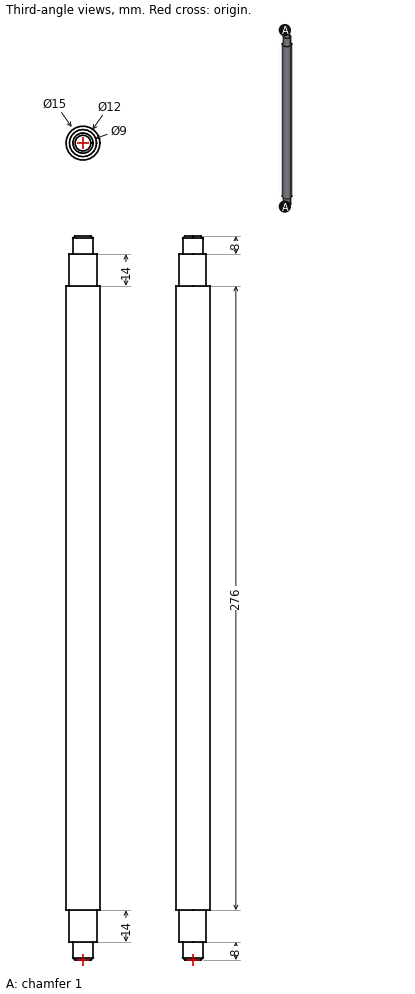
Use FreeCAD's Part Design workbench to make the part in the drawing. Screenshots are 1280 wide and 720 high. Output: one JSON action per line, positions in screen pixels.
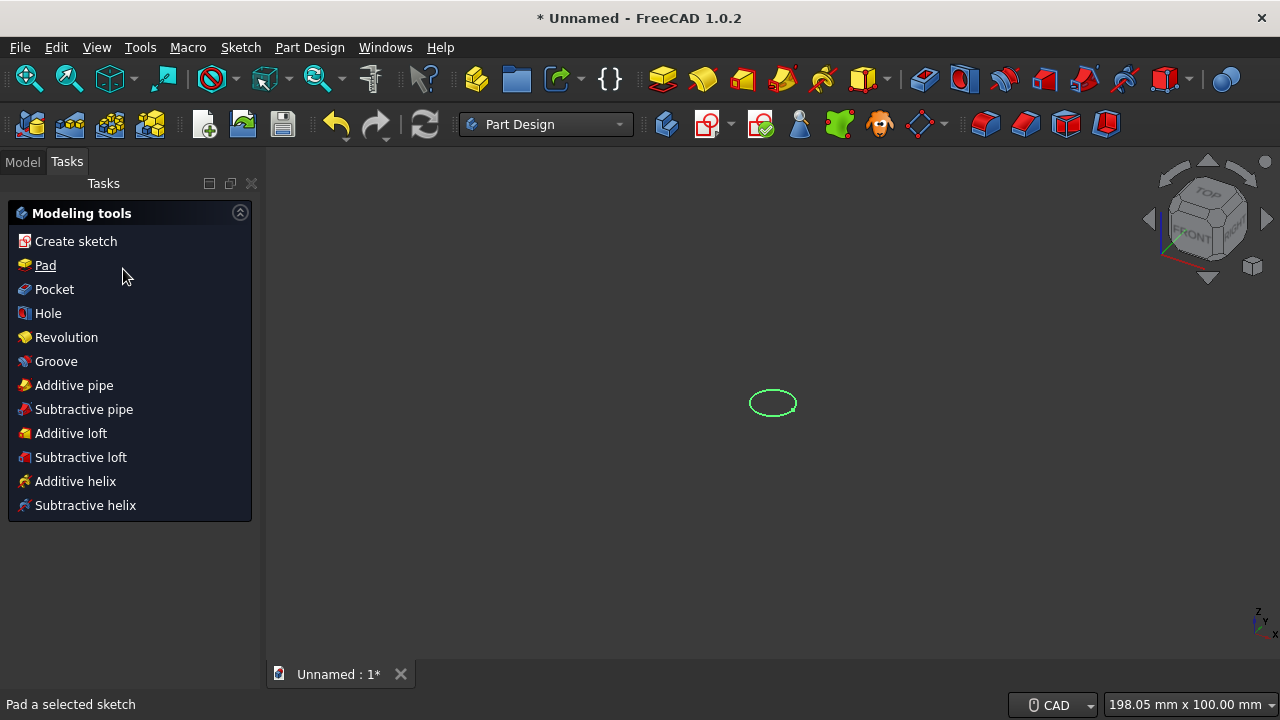
{"action": "left_click", "coordinate": [664, 80]}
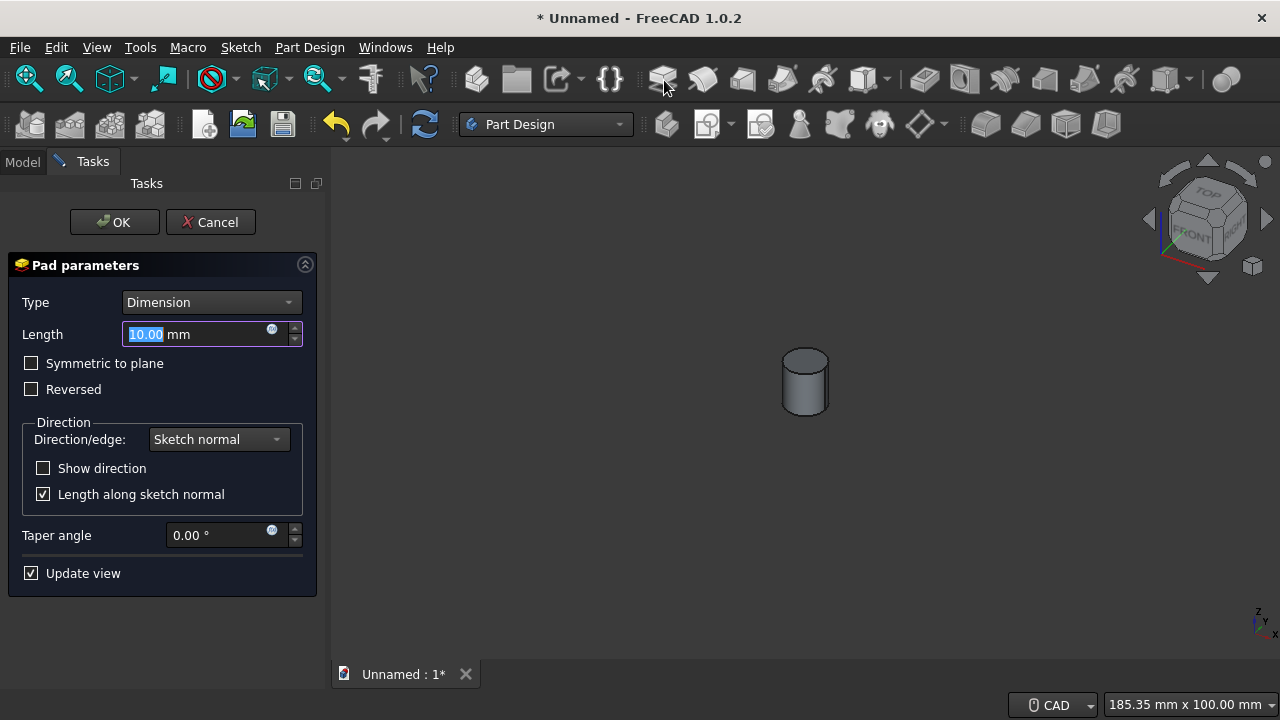
{"action": "type", "text": "8"}
{"action": "key", "text": "Tab"}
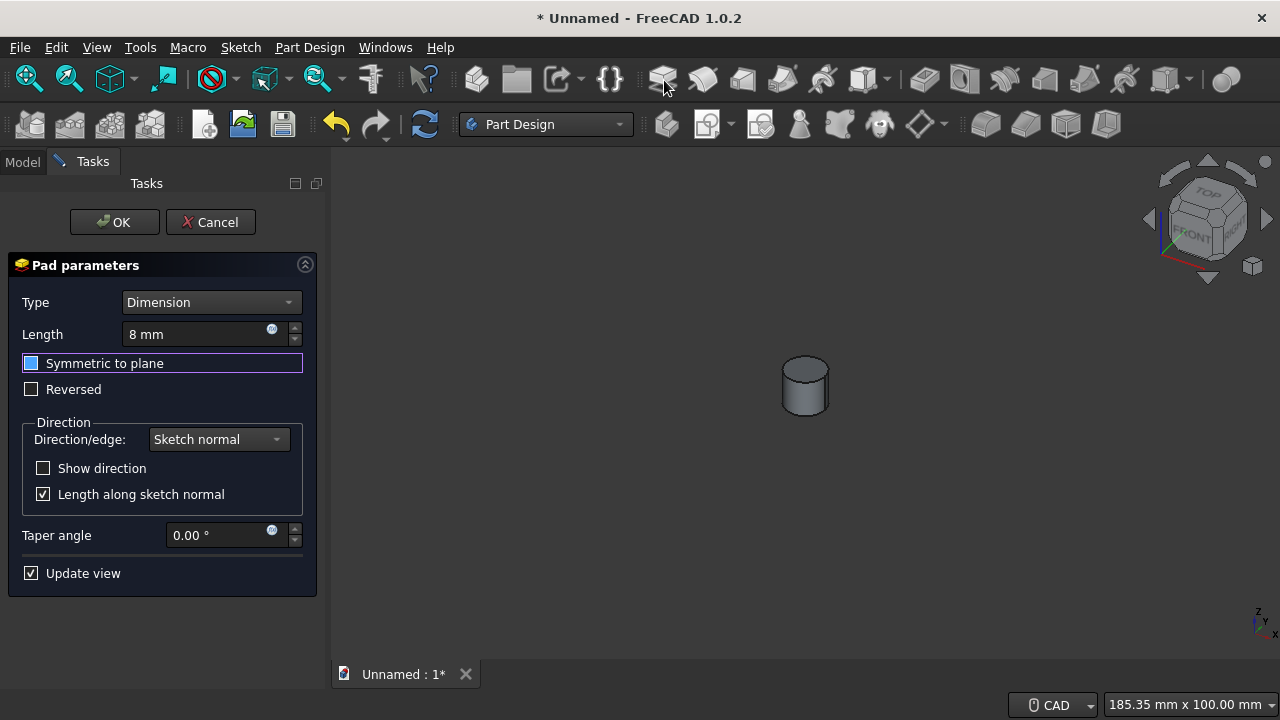
{"action": "left_click", "coordinate": [115, 222]}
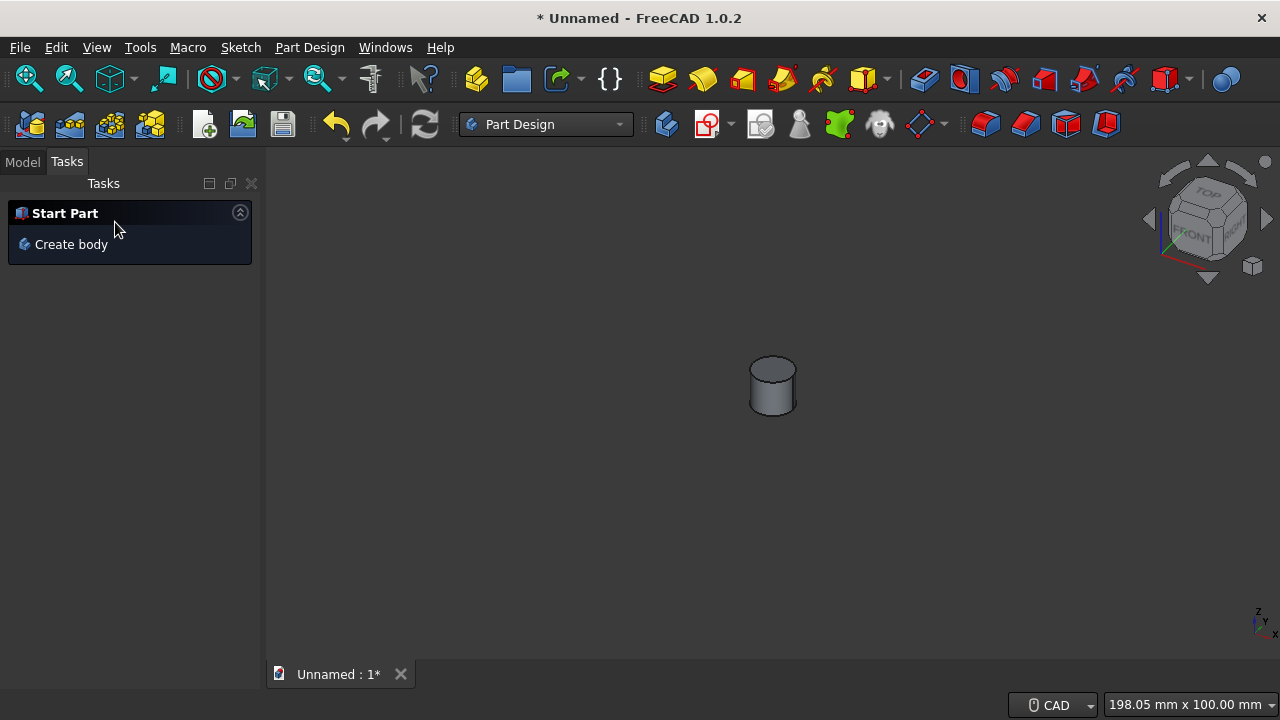
{"action": "key", "text": "v f"}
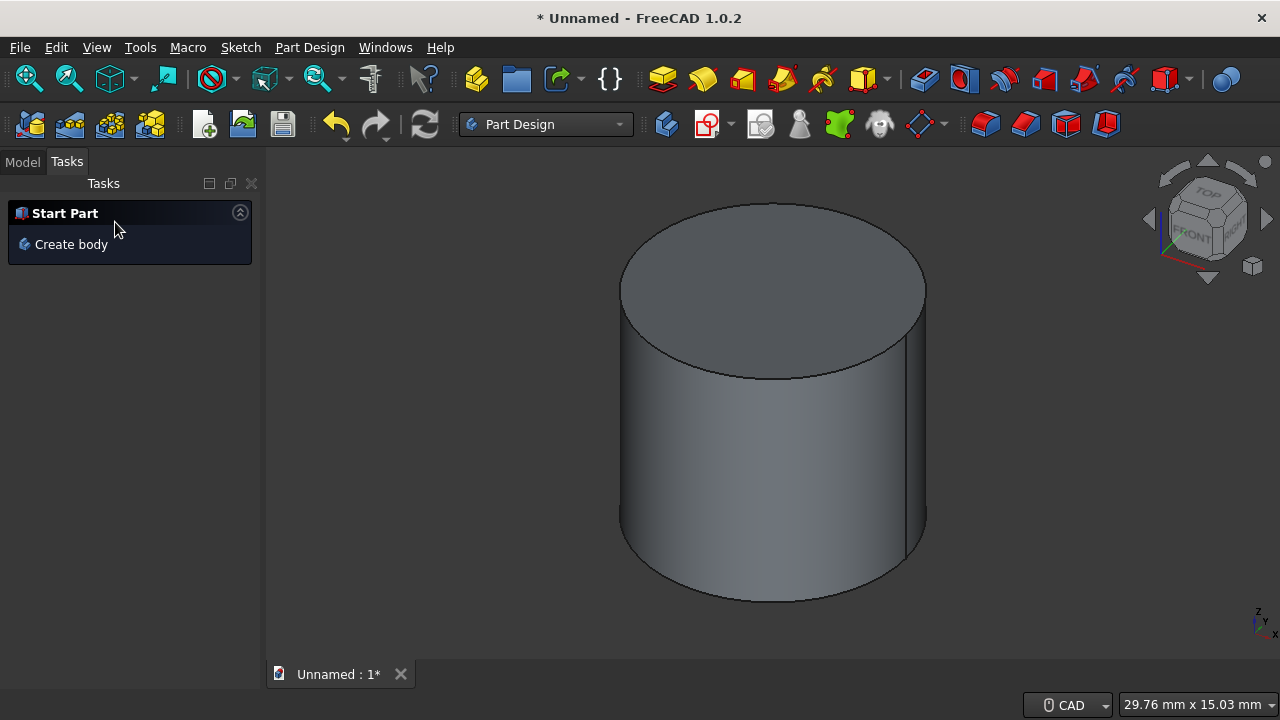
{"action": "left_click", "coordinate": [773, 290]}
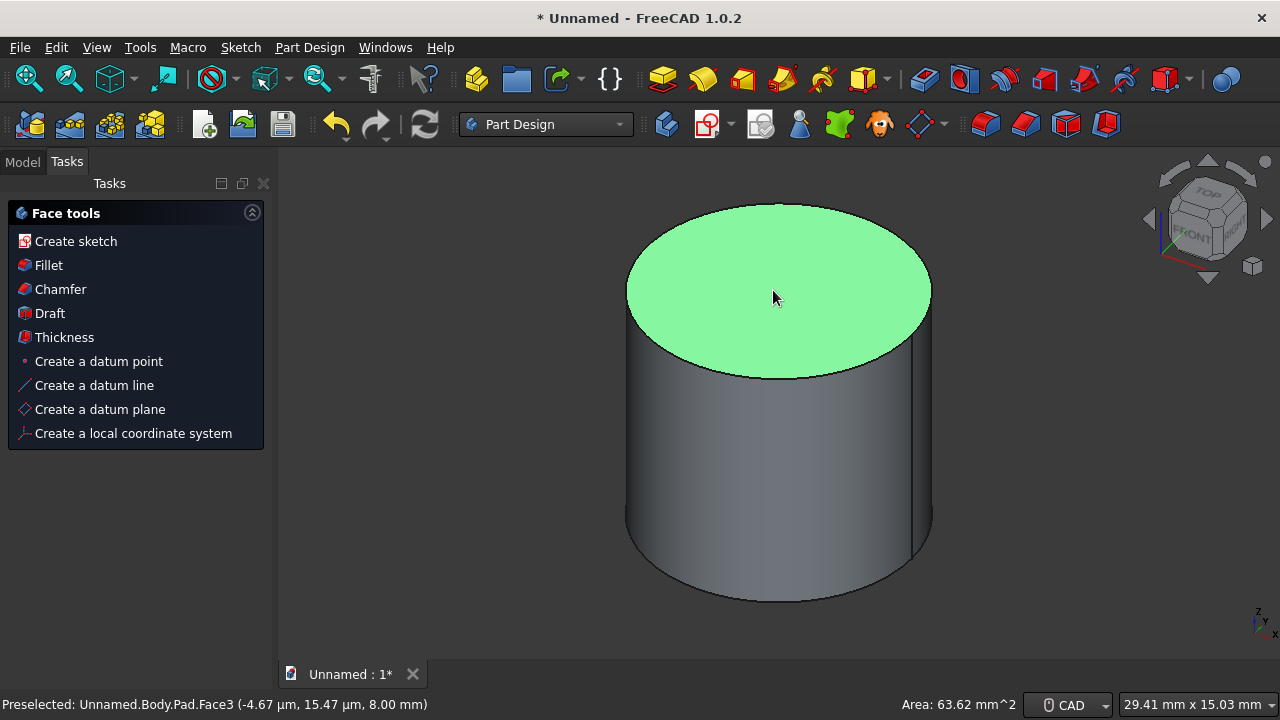
{"action": "left_click", "coordinate": [708, 124]}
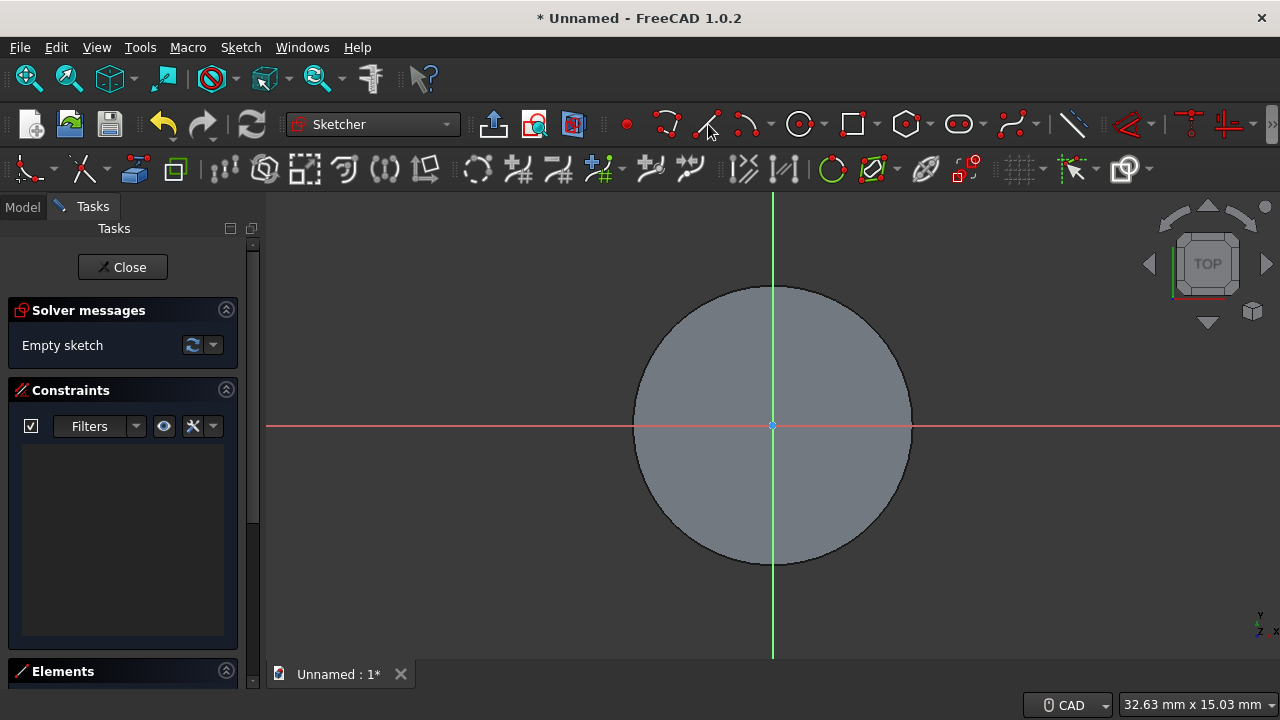
{"action": "scroll", "coordinate": [396, 425], "scroll_direction": "down", "scroll_amount": 1}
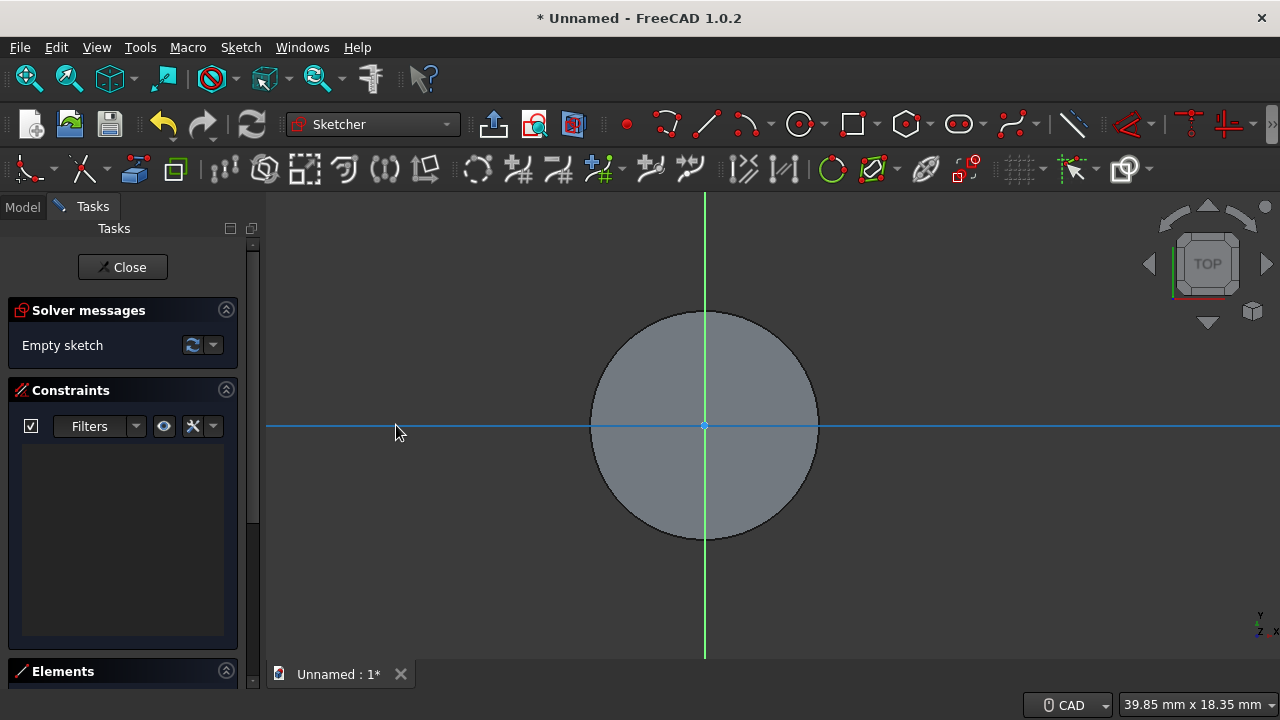
{"action": "key", "text": "g c"}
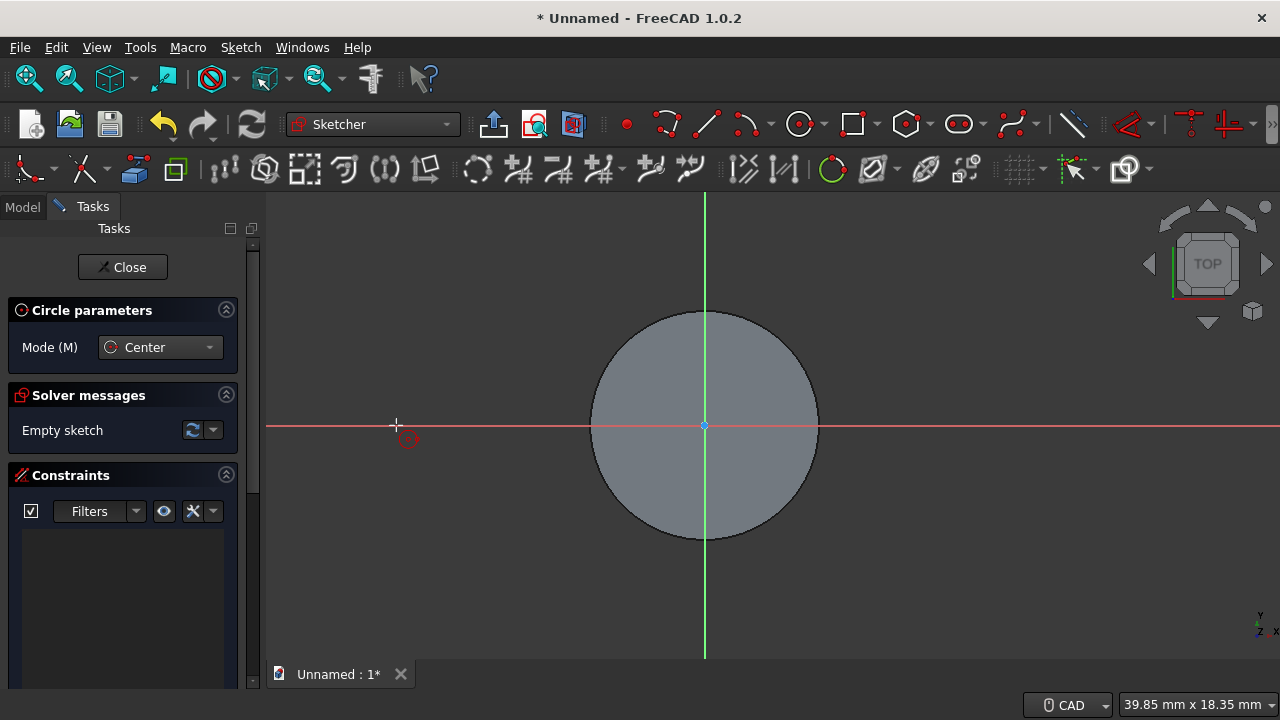
{"action": "left_click", "coordinate": [705, 426]}
{"action": "left_click", "coordinate": [813, 318]}
{"action": "key", "text": "Escape"}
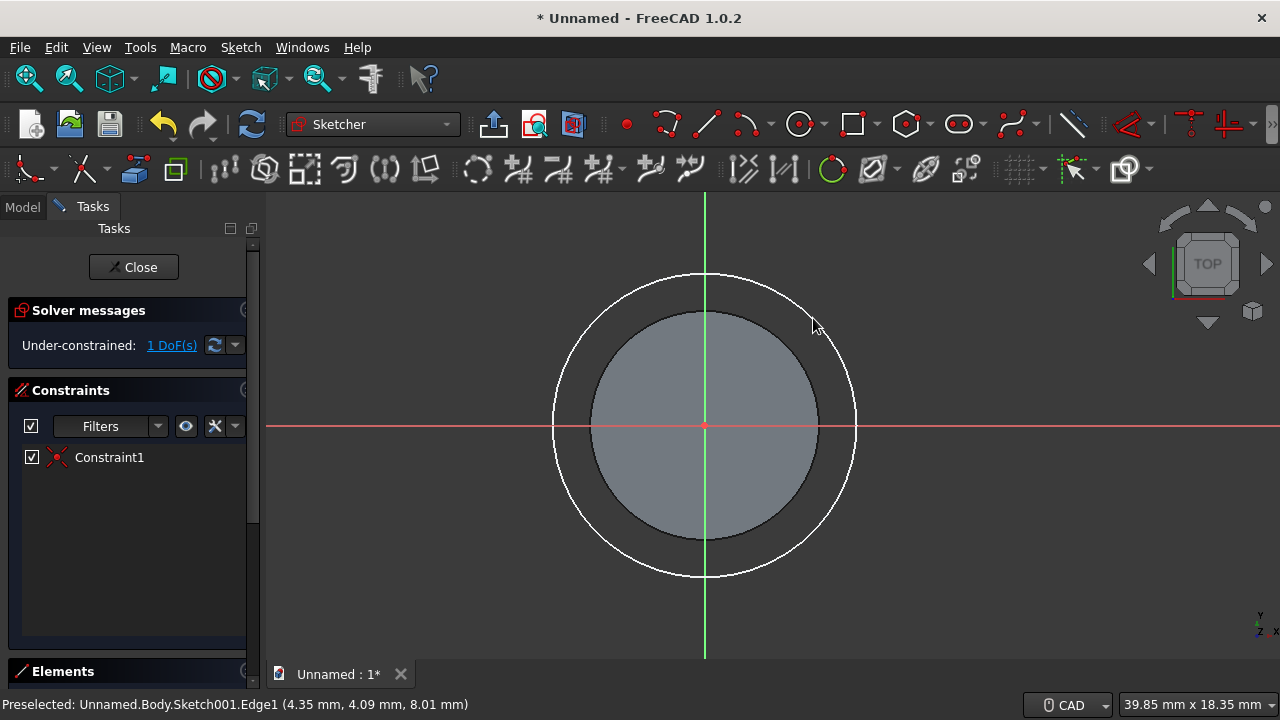
{"action": "left_click", "coordinate": [1128, 124]}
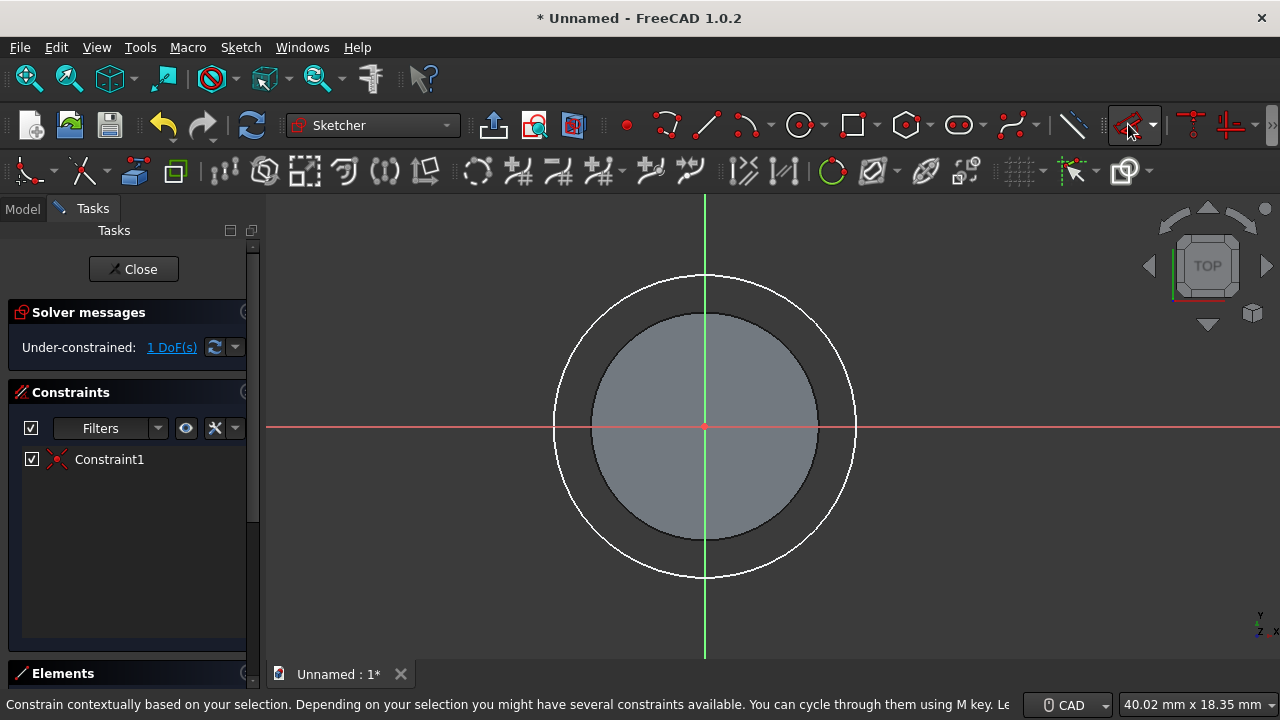
{"action": "left_click", "coordinate": [812, 319]}
{"action": "left_click", "coordinate": [835, 296]}